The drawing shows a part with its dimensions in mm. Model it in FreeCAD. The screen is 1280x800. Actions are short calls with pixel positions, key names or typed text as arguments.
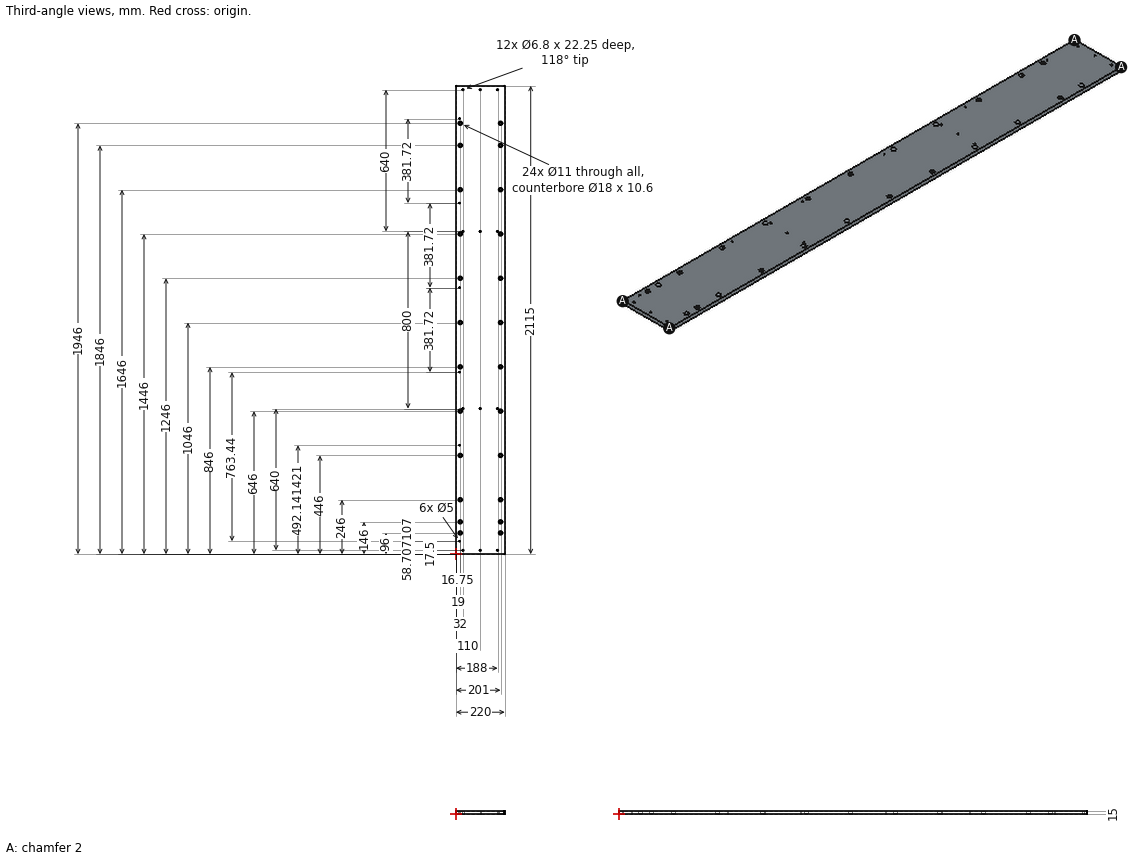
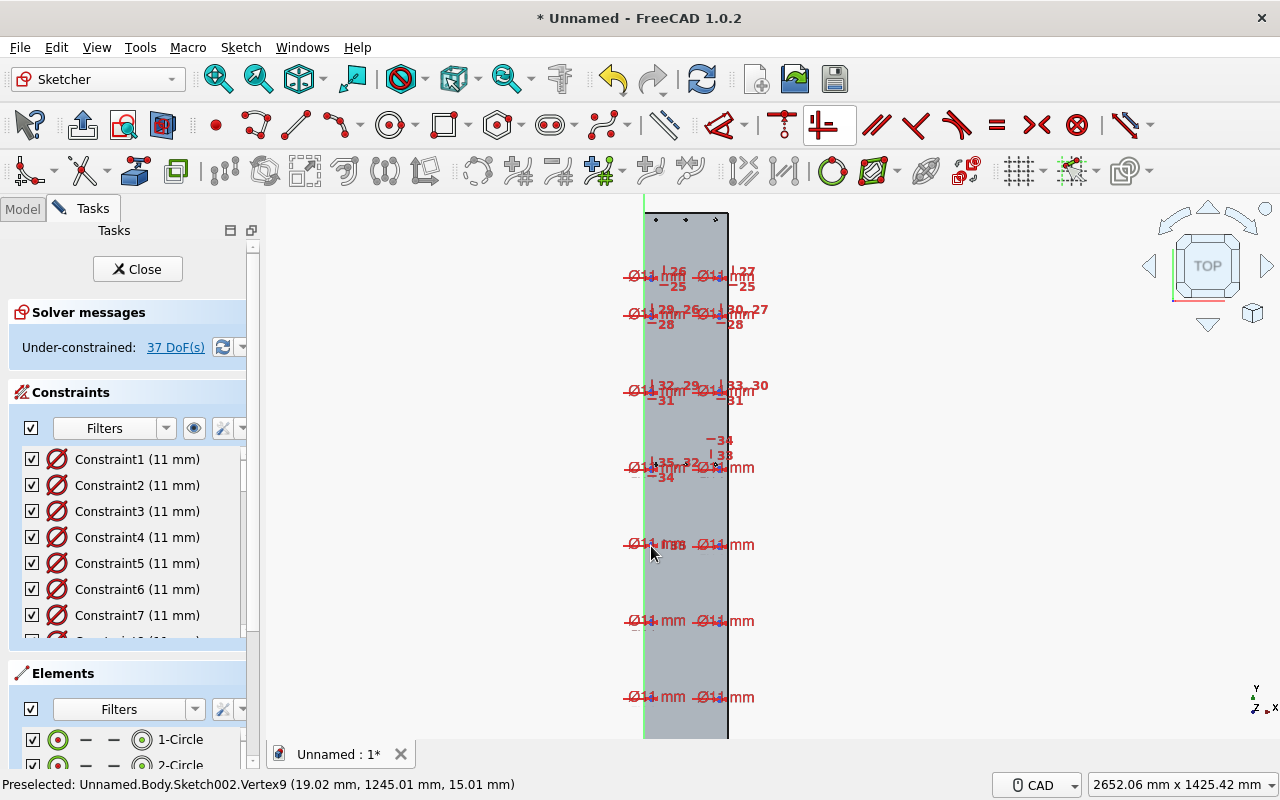
click(720, 470)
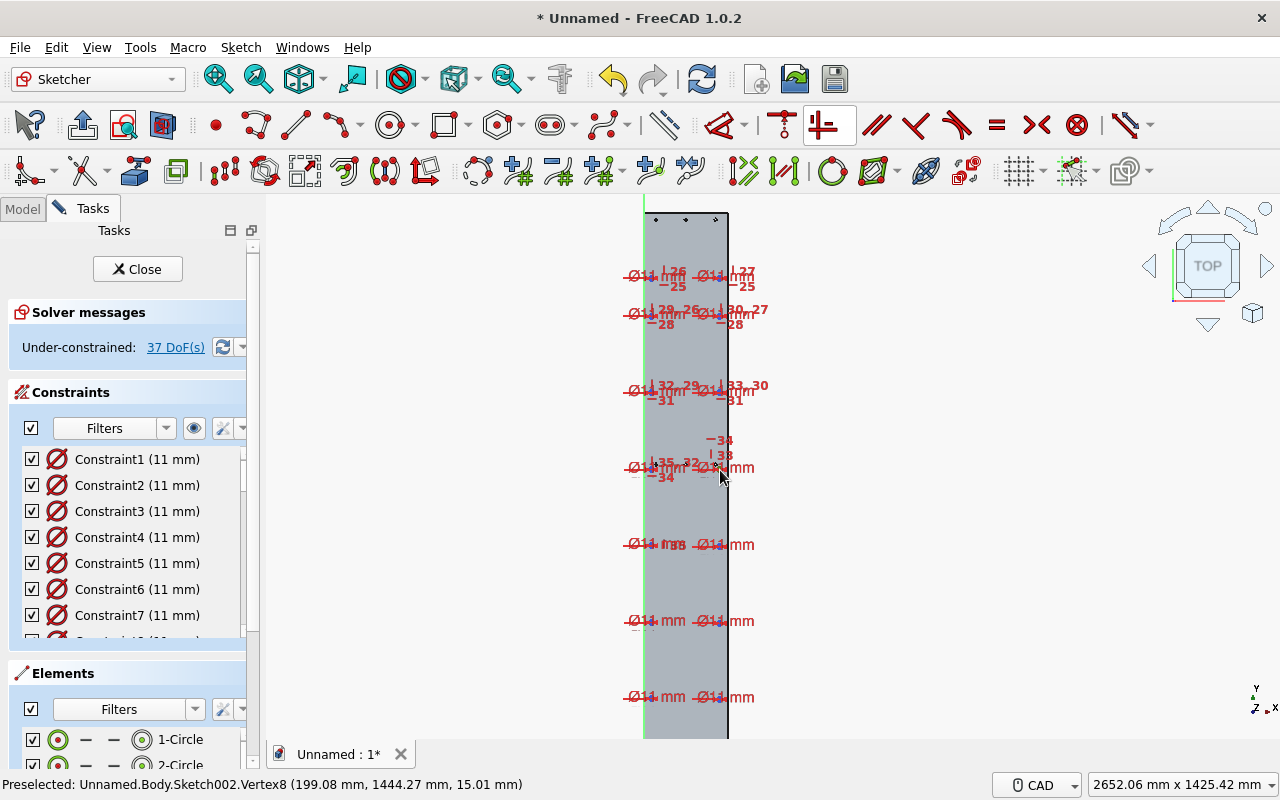
click(720, 547)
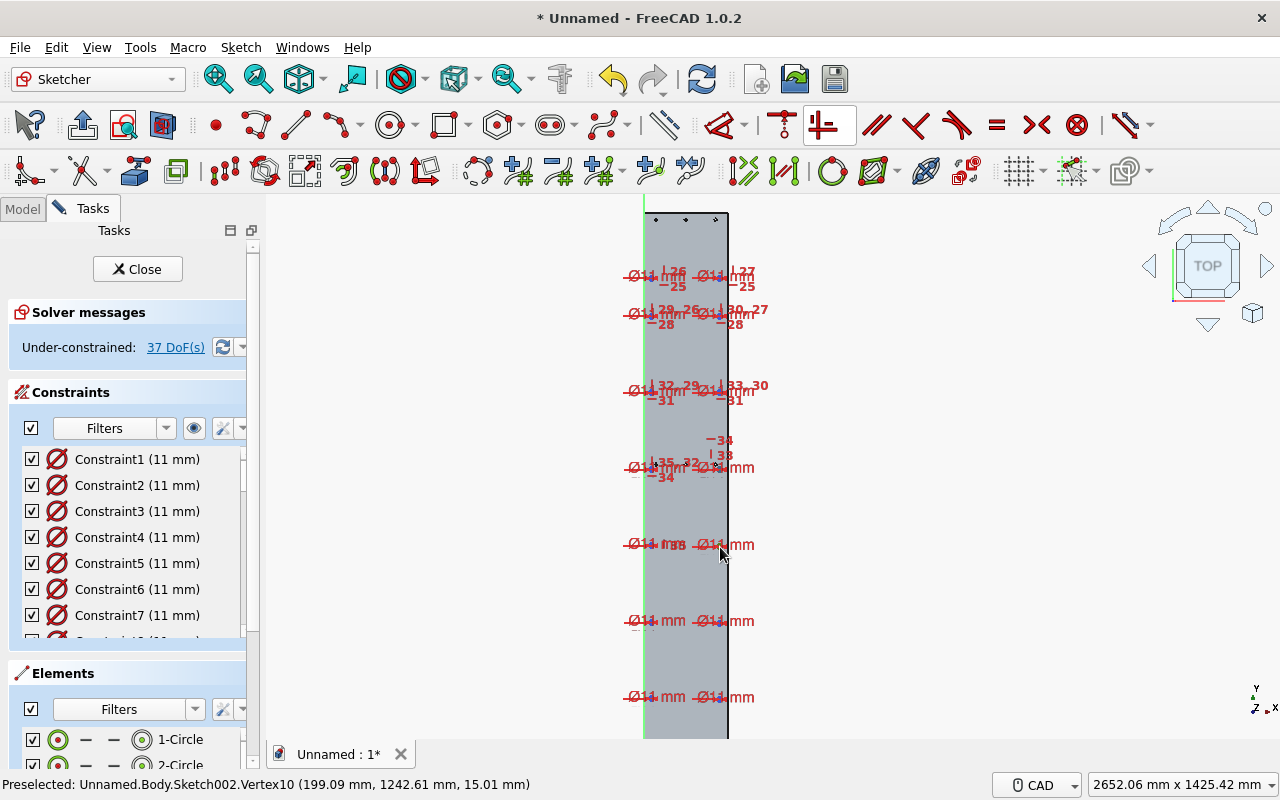
click(850, 126)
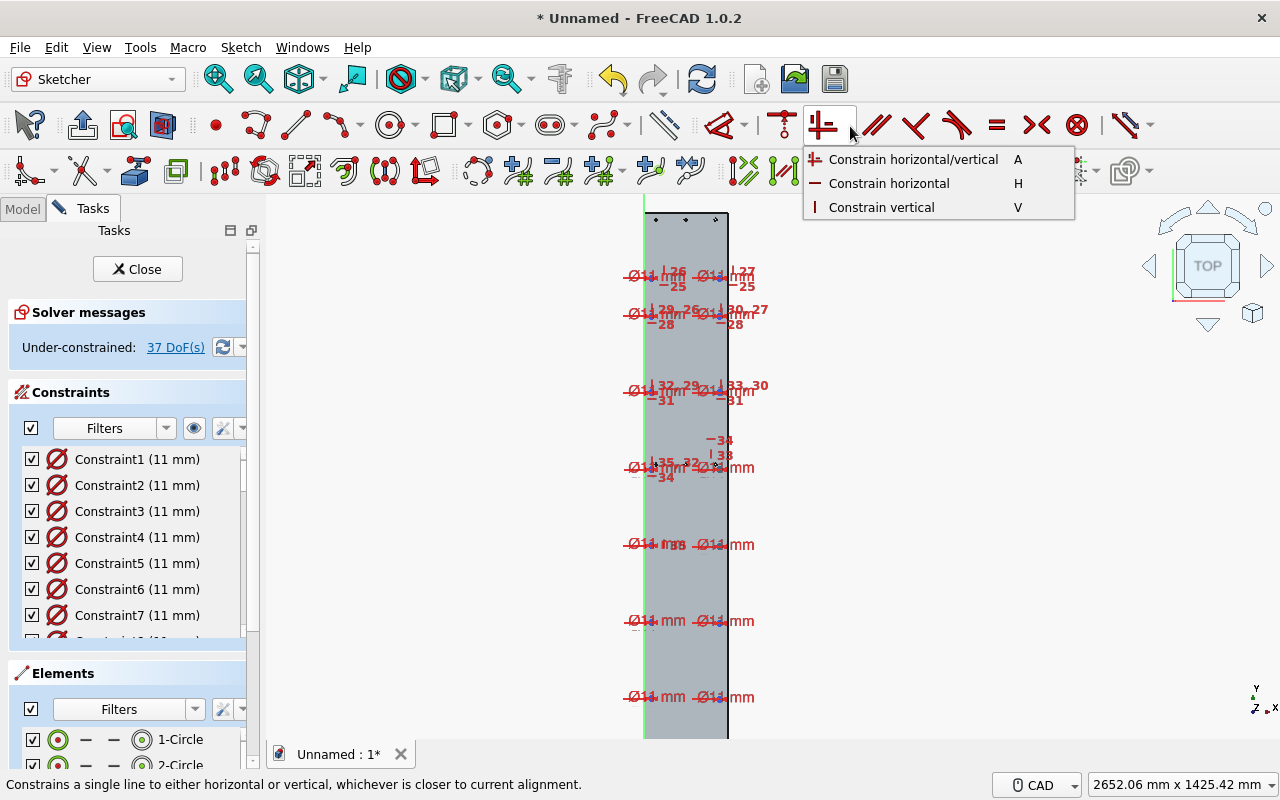
click(939, 207)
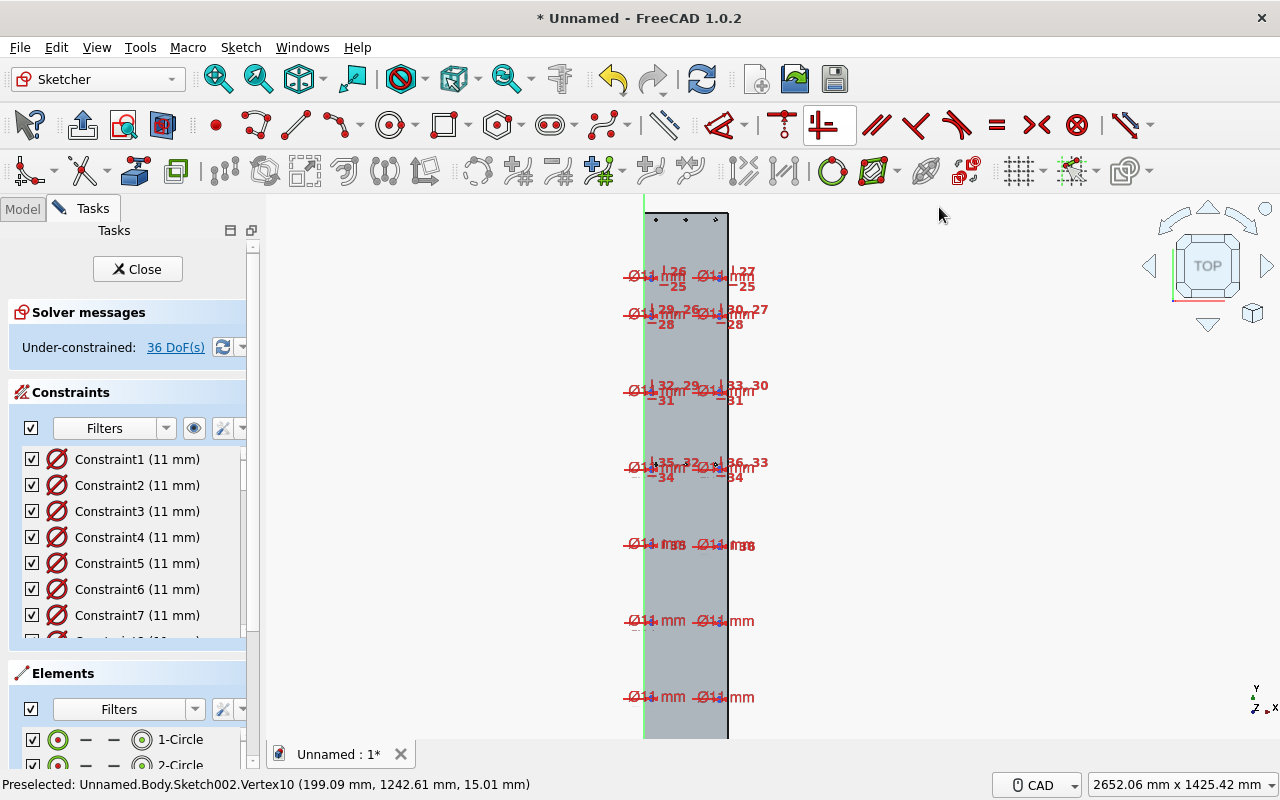
click(651, 546)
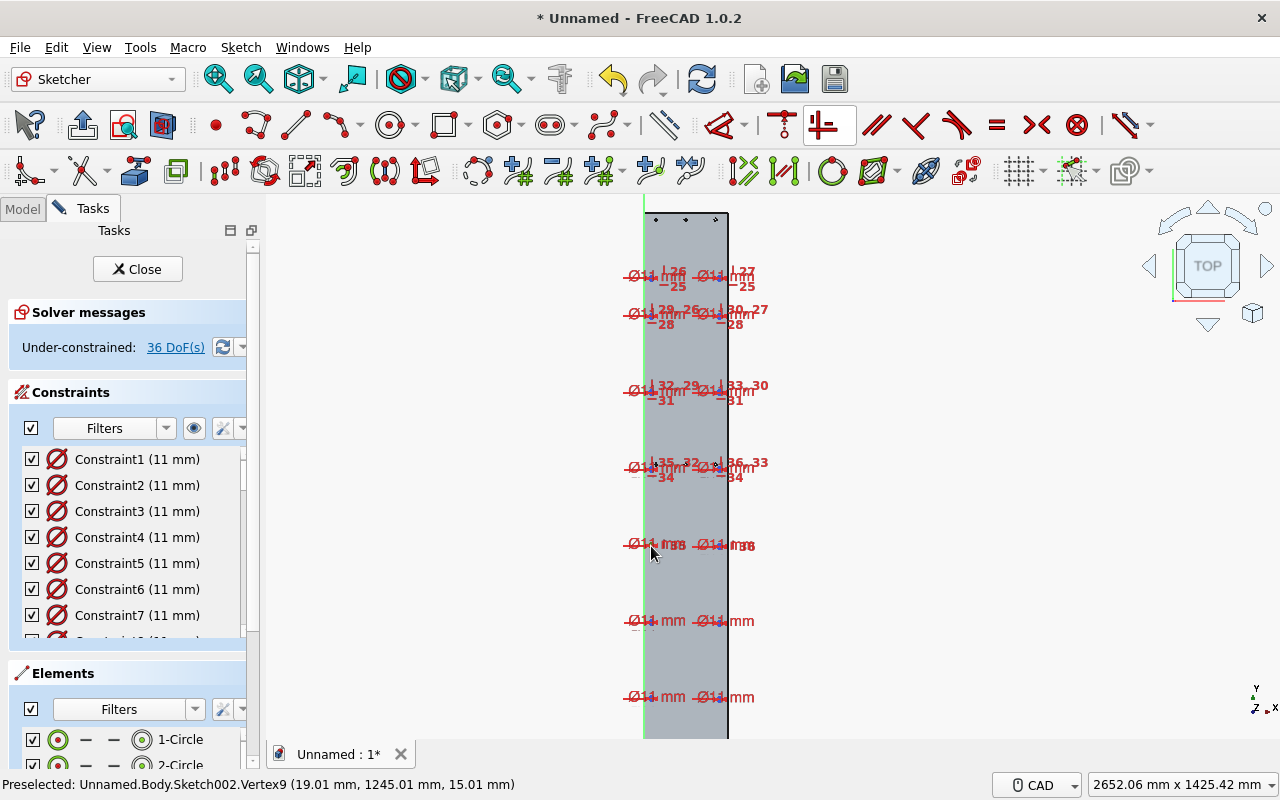
click(720, 547)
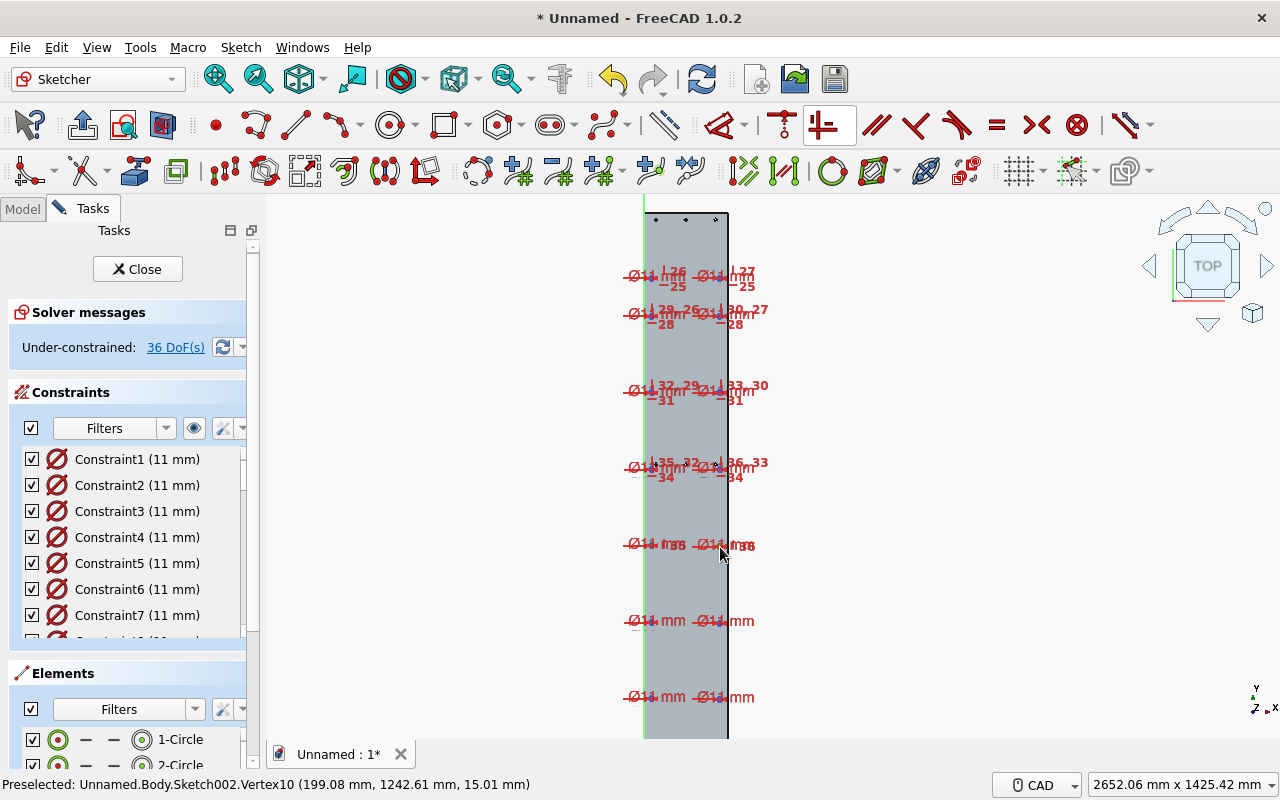
key(h)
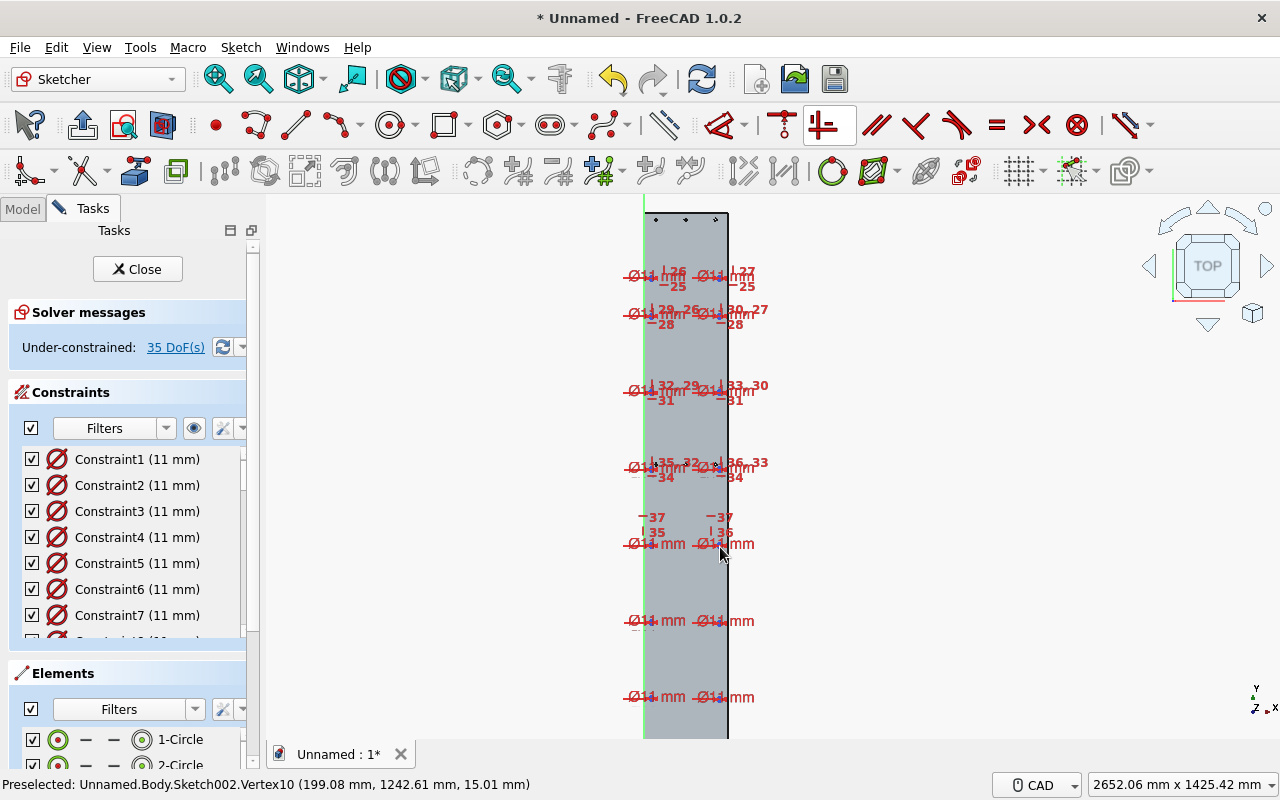
click(651, 546)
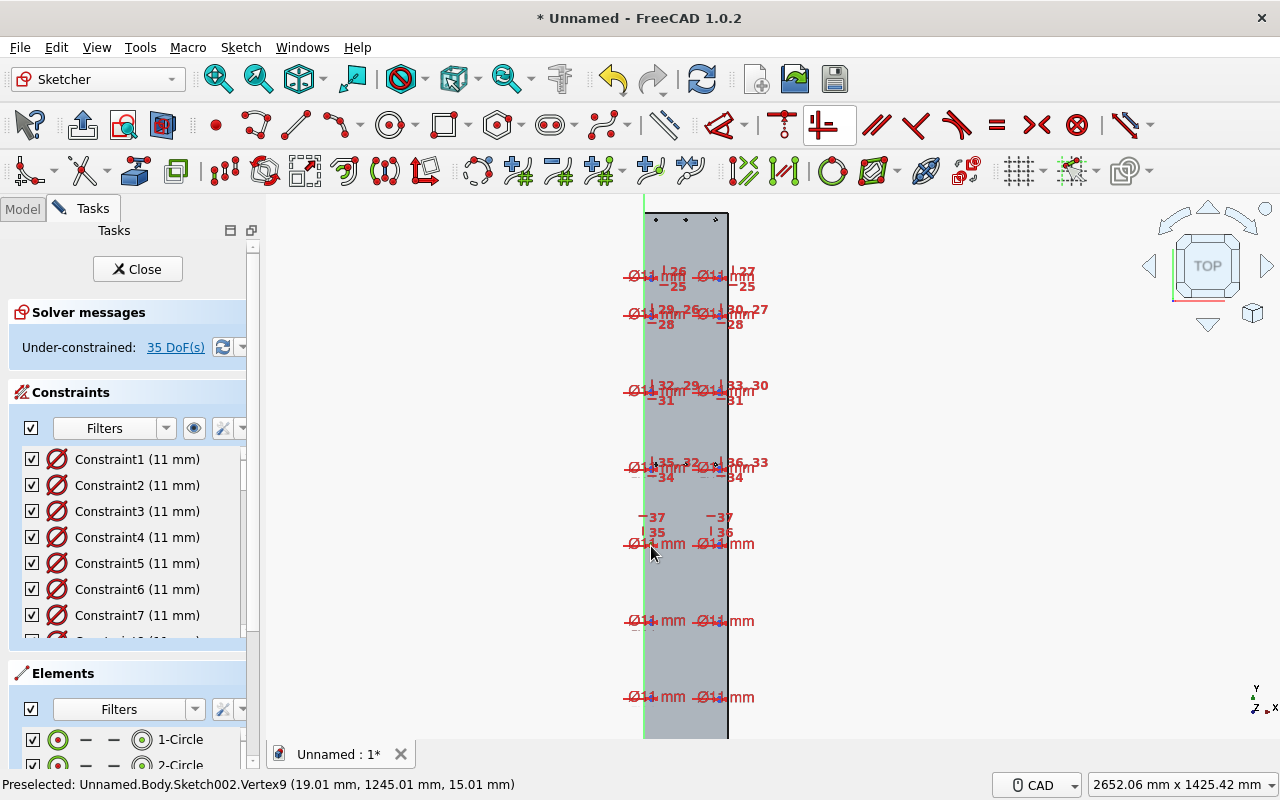
click(651, 623)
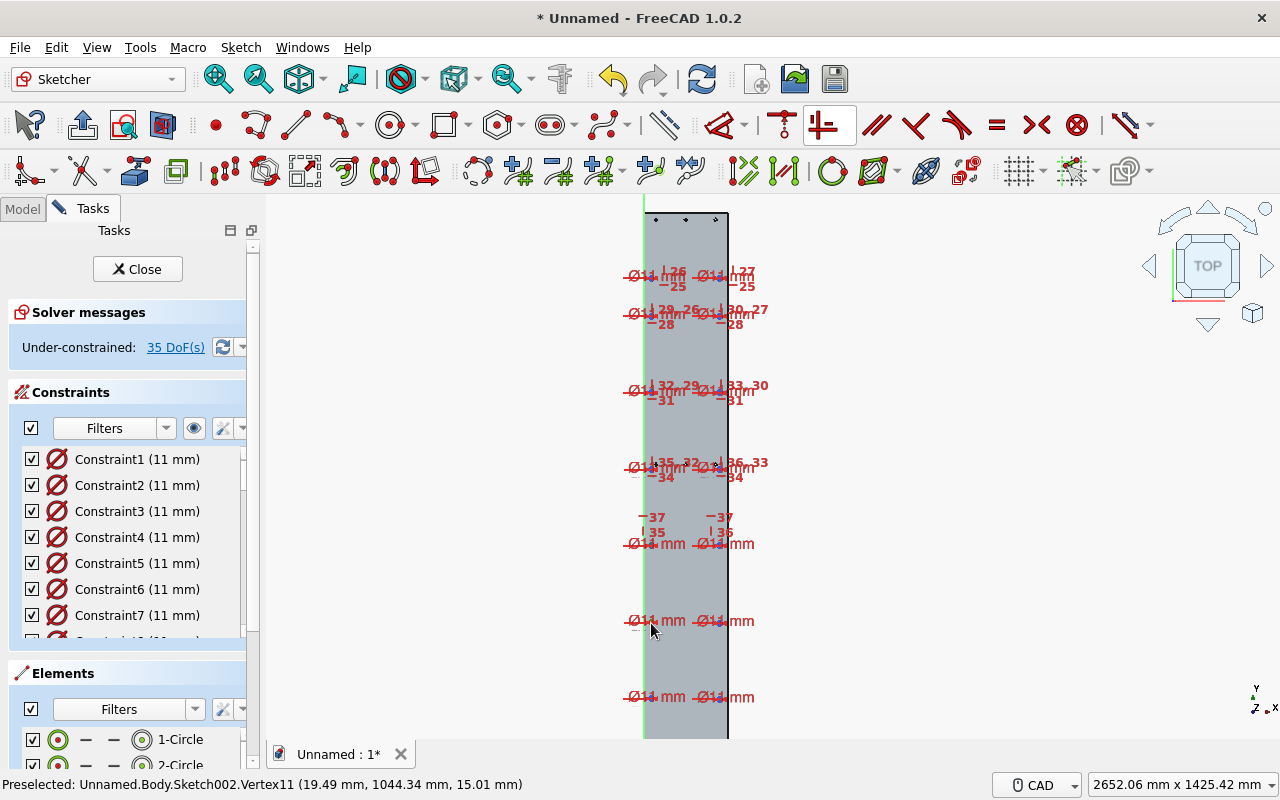
click(850, 126)